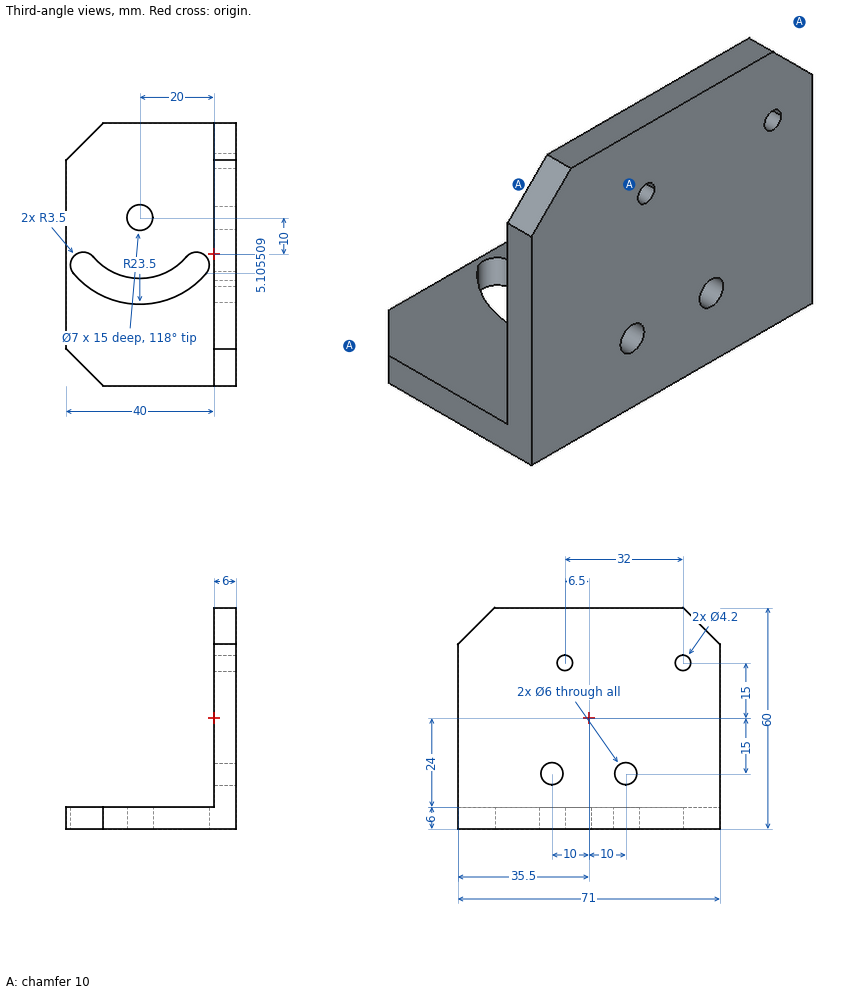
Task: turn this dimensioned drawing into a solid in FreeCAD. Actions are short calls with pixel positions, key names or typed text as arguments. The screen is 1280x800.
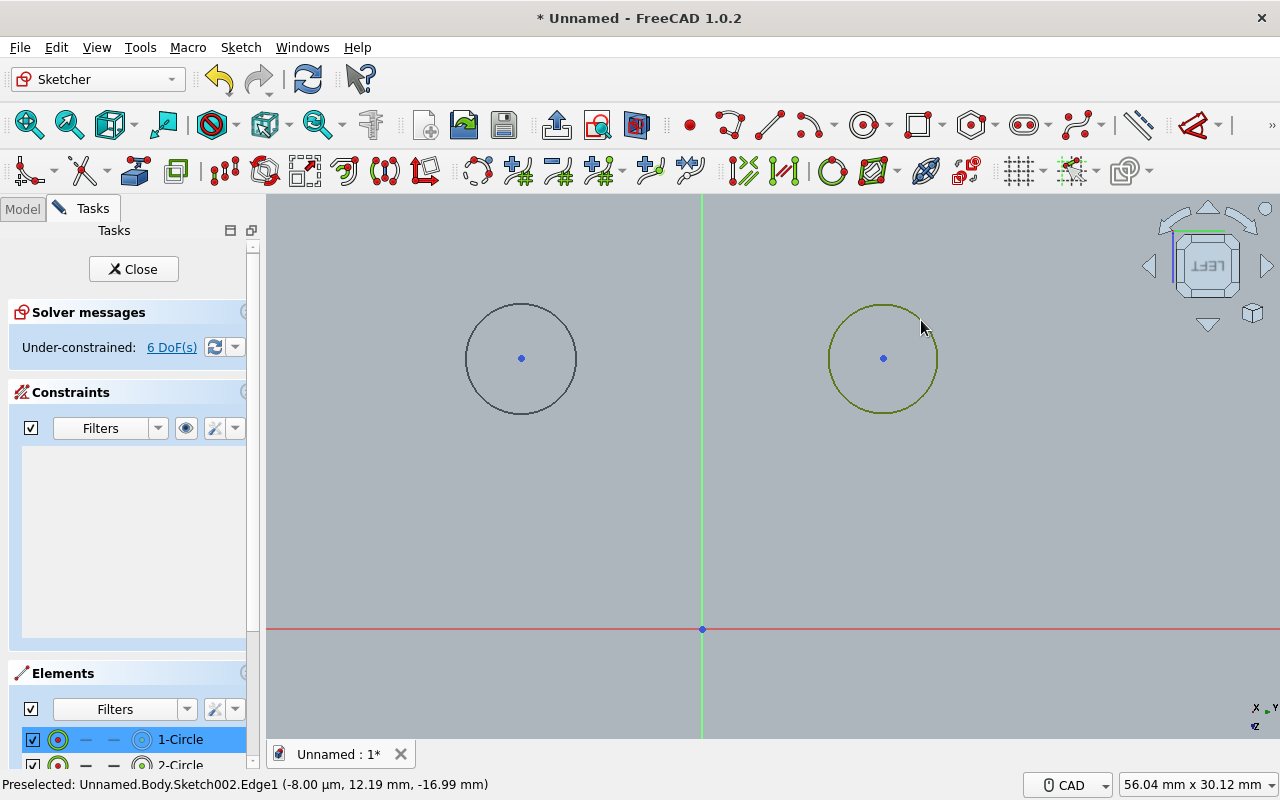
click(560, 320)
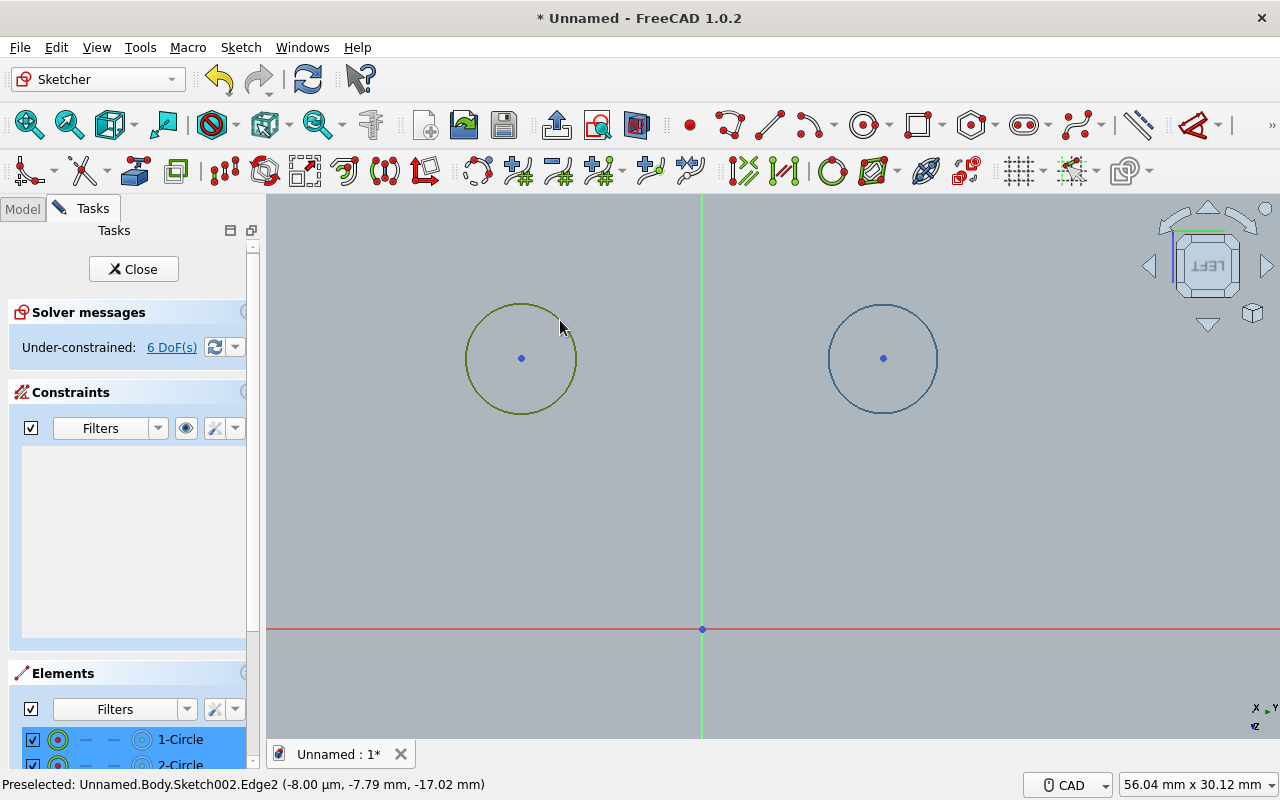
key(e)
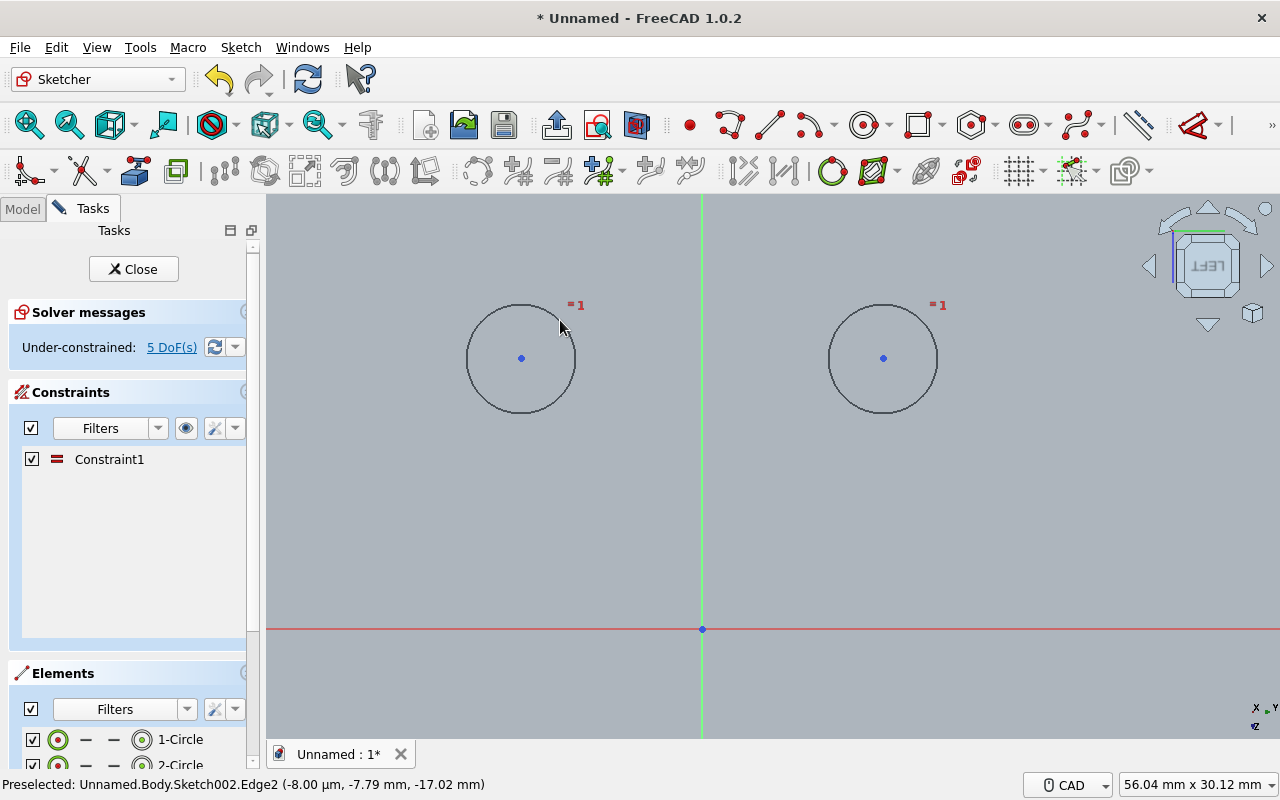
click(883, 359)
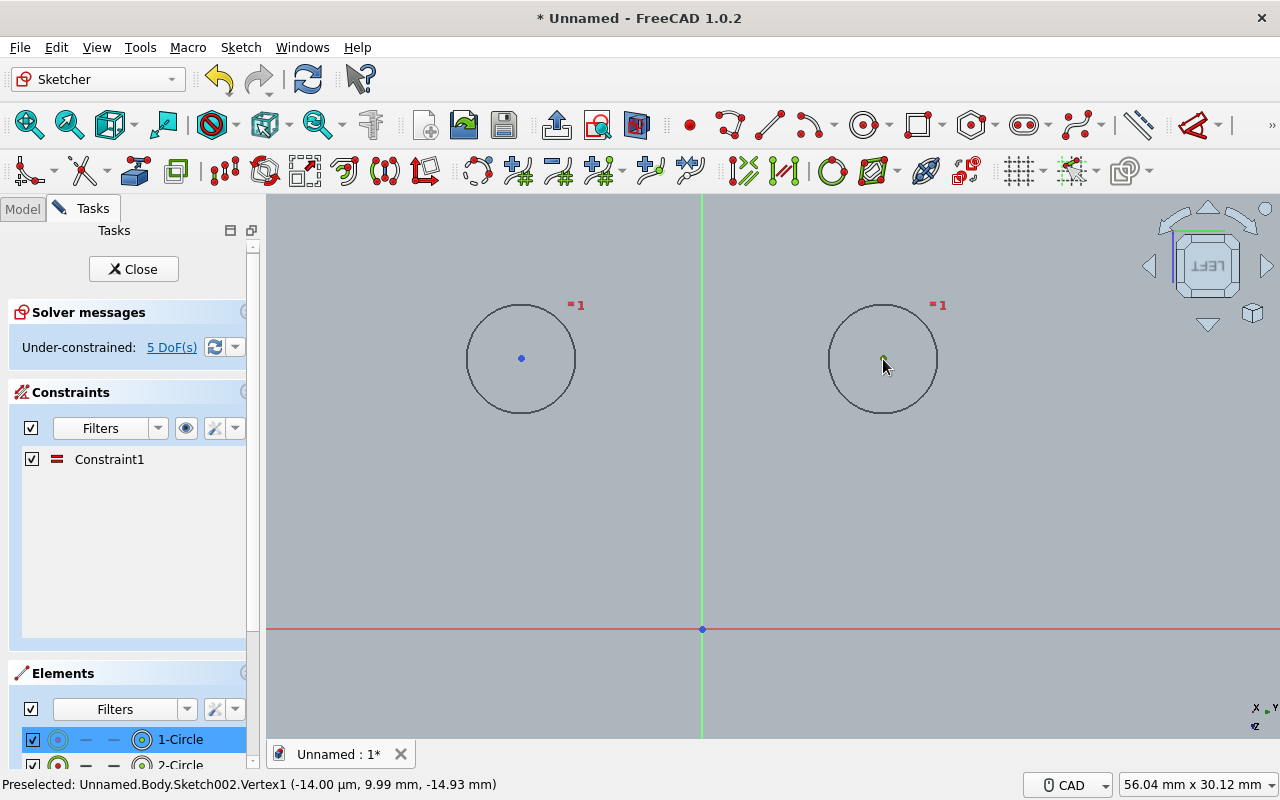
click(521, 359)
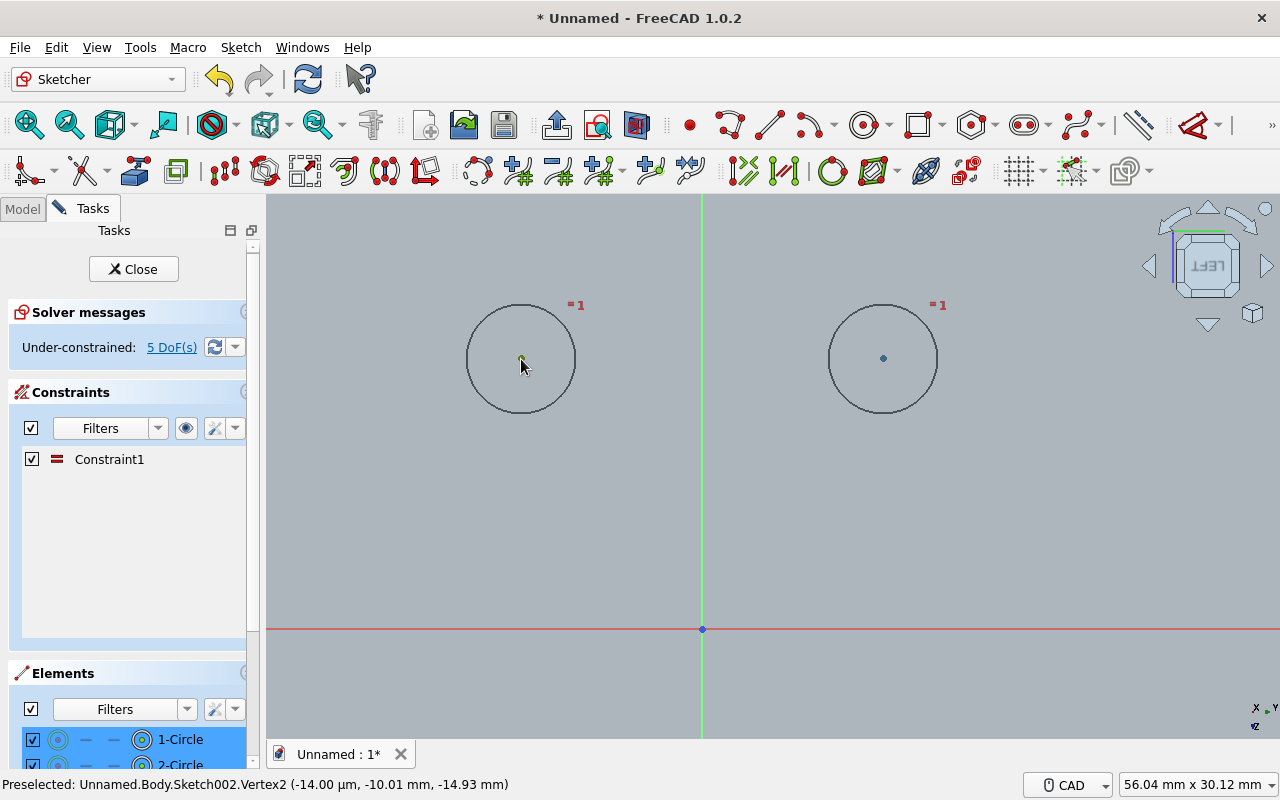
key(h)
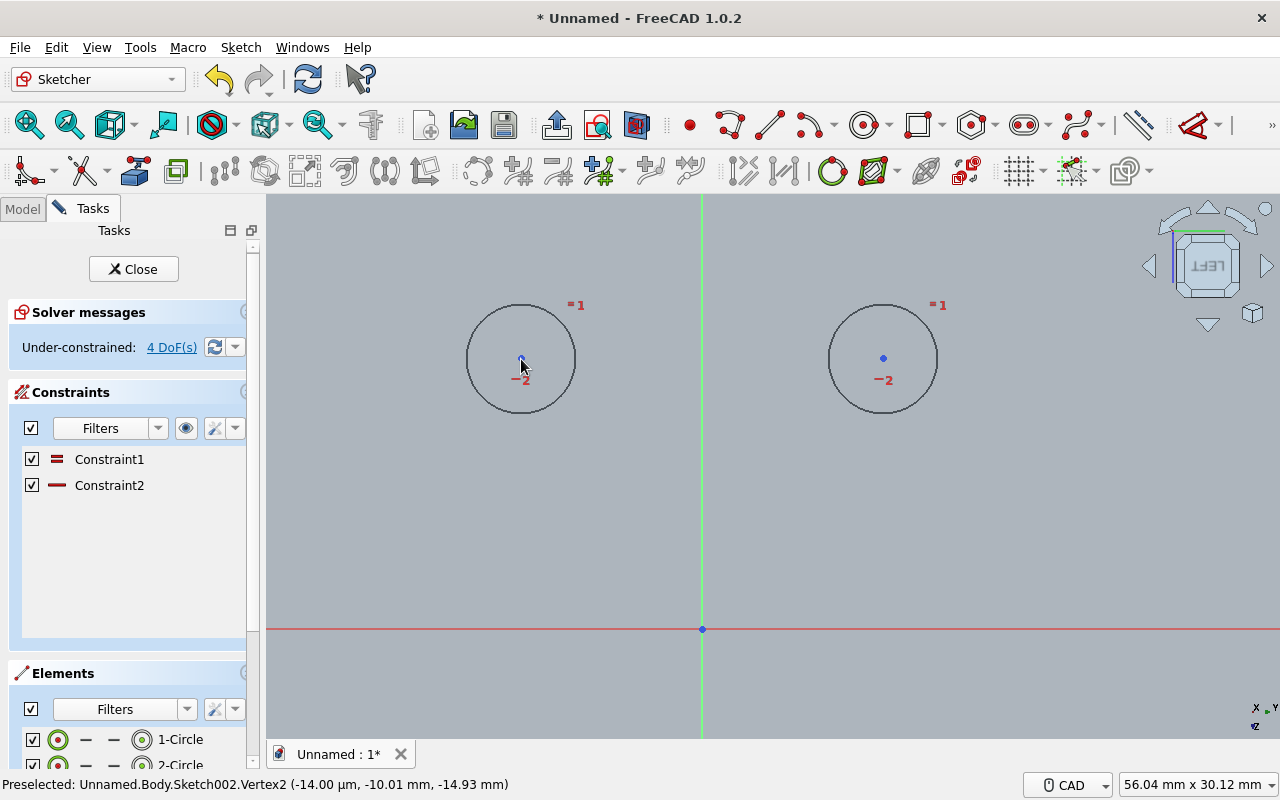
click(1194, 126)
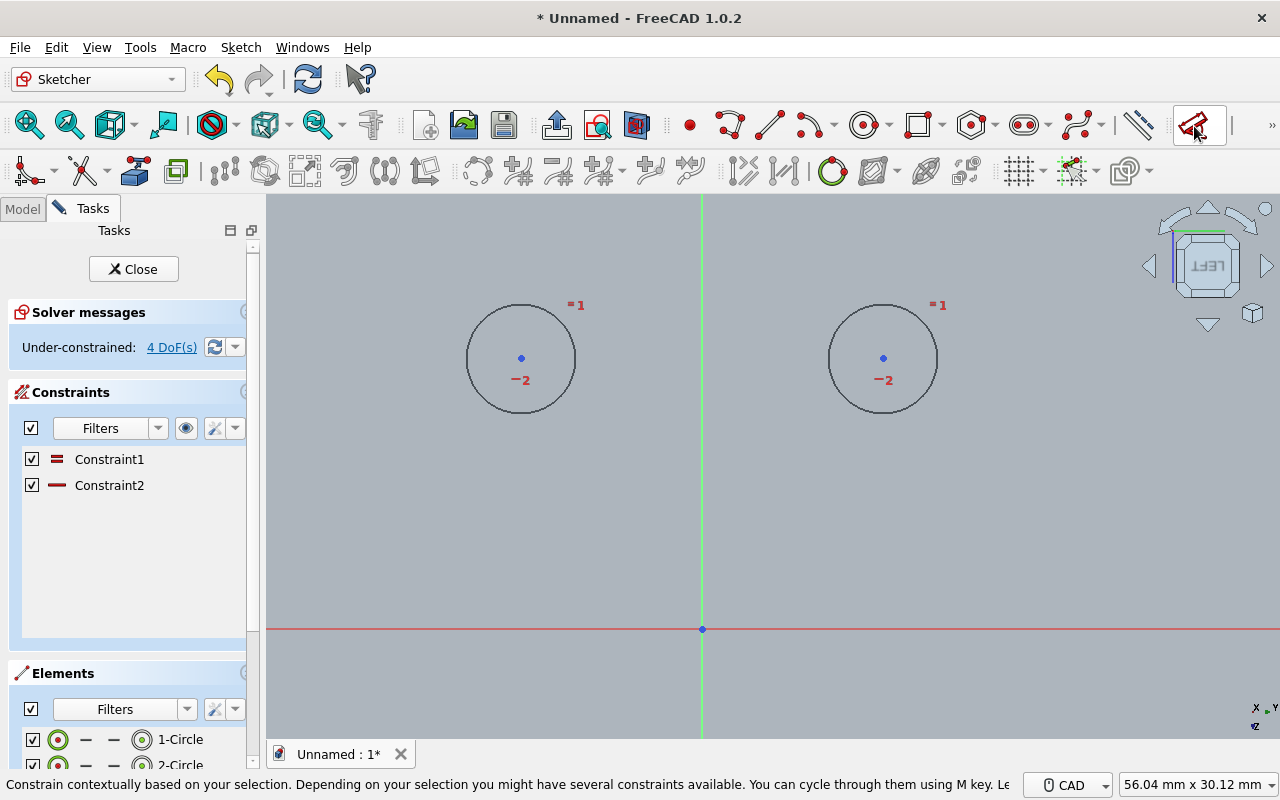
click(921, 320)
click(943, 297)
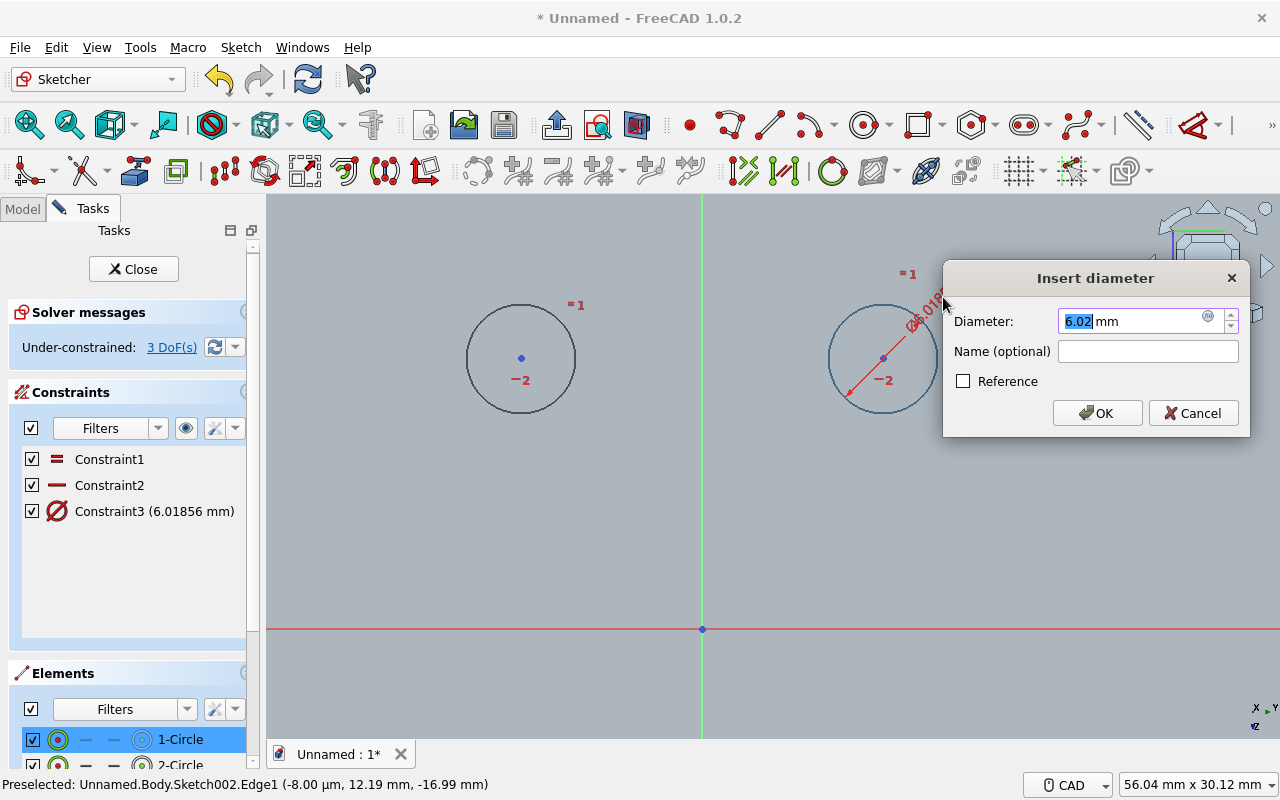
text(6)
key(Return)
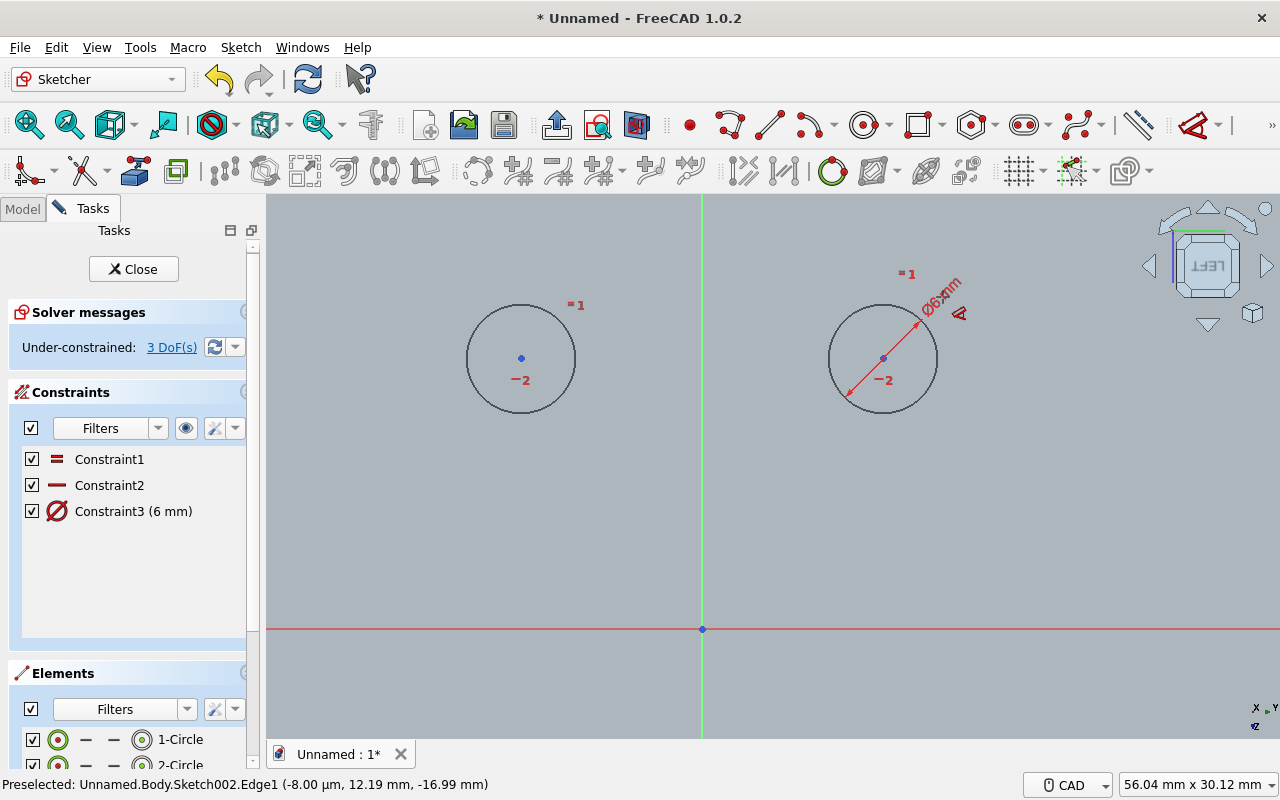
click(883, 359)
click(793, 663)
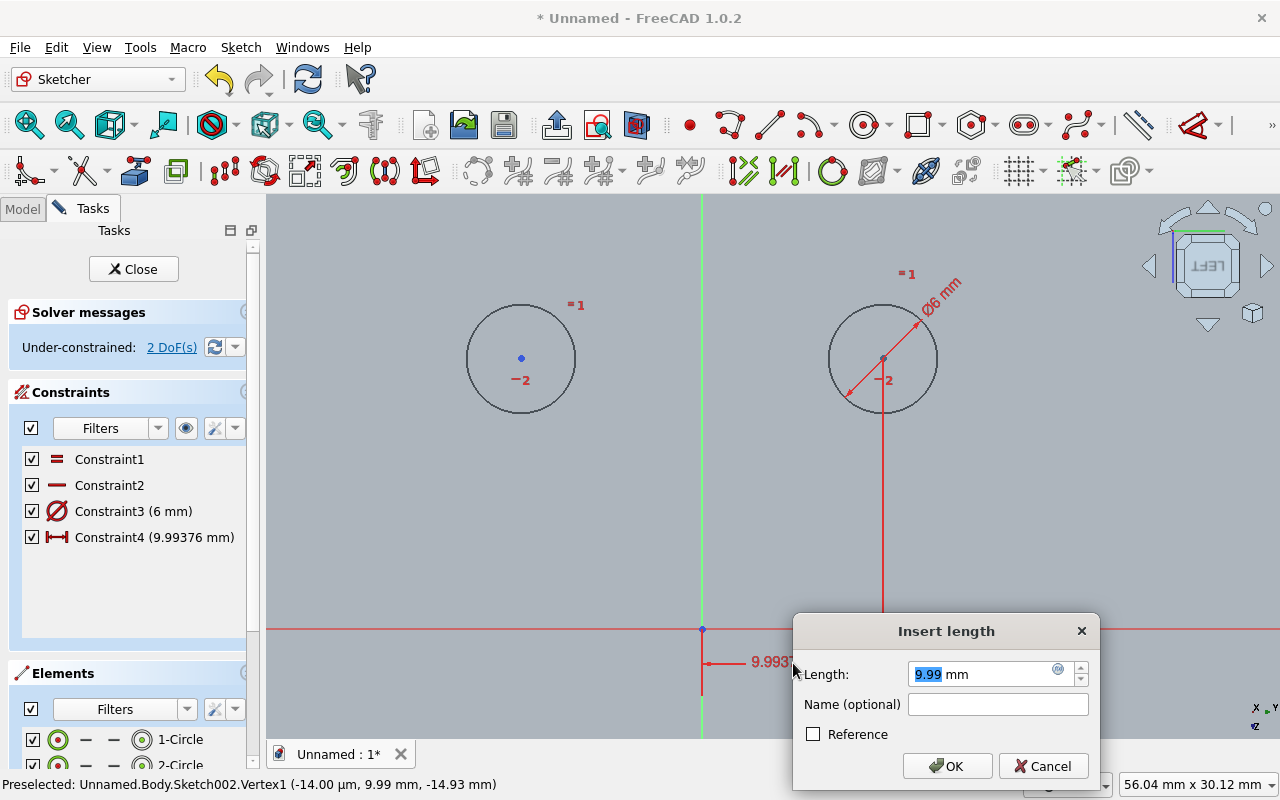
text(10)
key(Return)